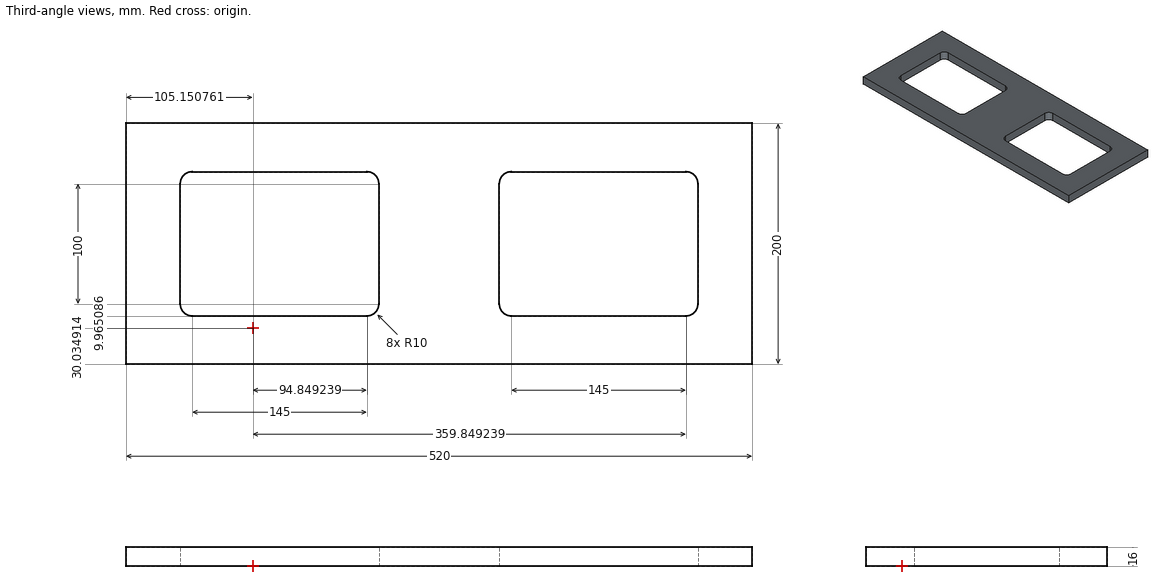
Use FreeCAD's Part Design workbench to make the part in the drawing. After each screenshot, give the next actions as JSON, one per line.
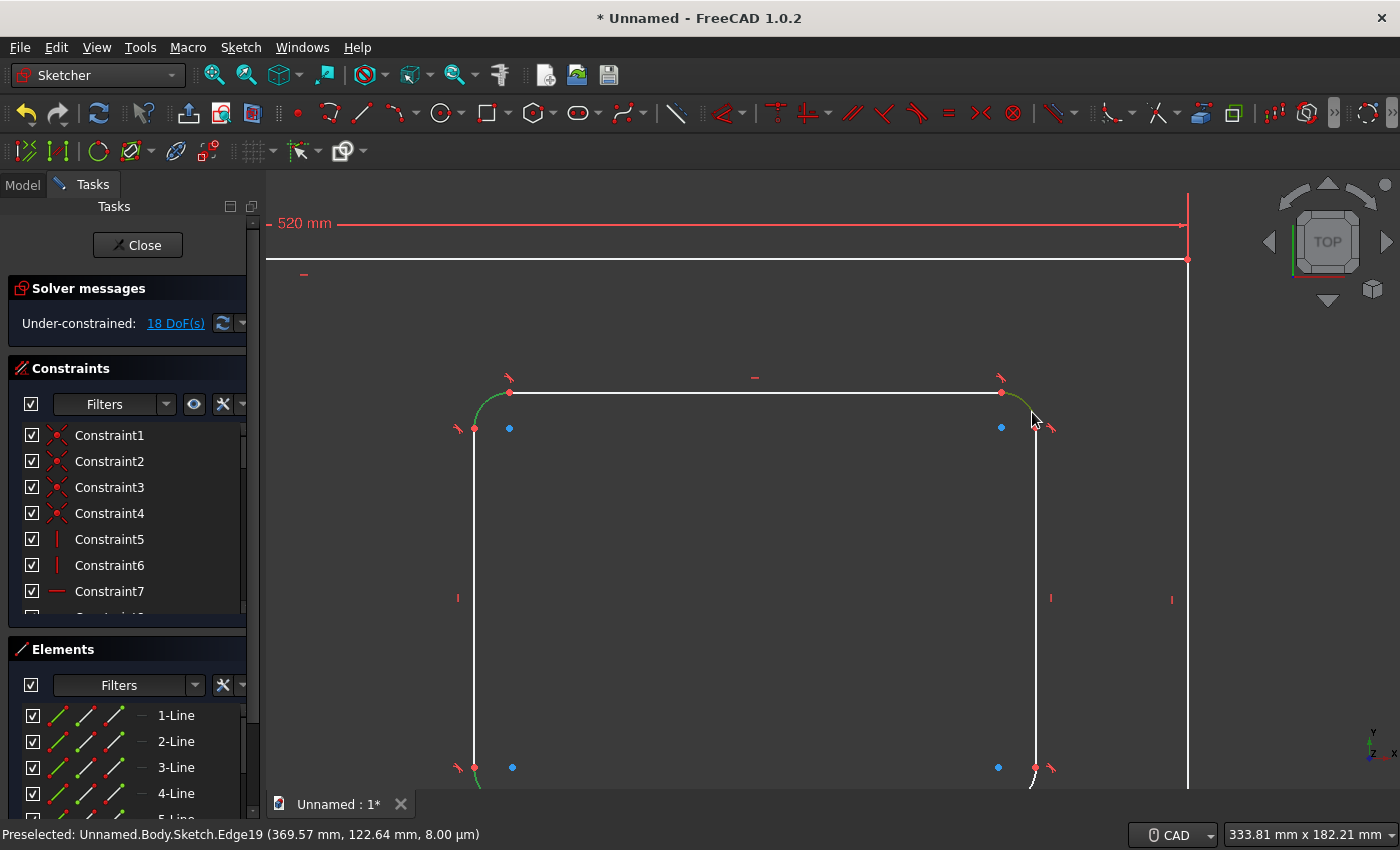
{"action": "scroll", "coordinate": [1032, 412], "scroll_direction": "down", "scroll_amount": 5}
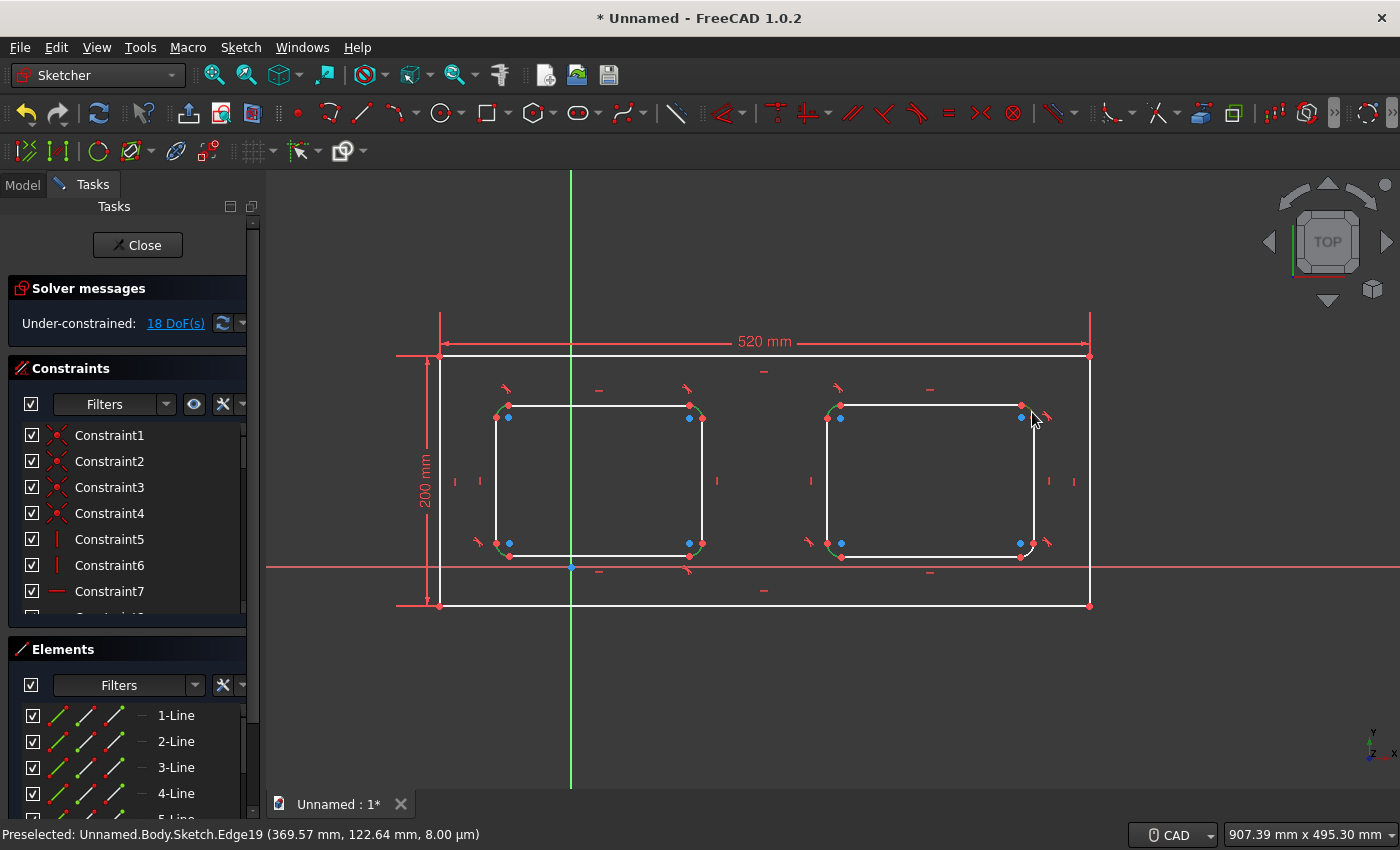
{"action": "scroll", "coordinate": [1026, 556], "scroll_direction": "up", "scroll_amount": 4}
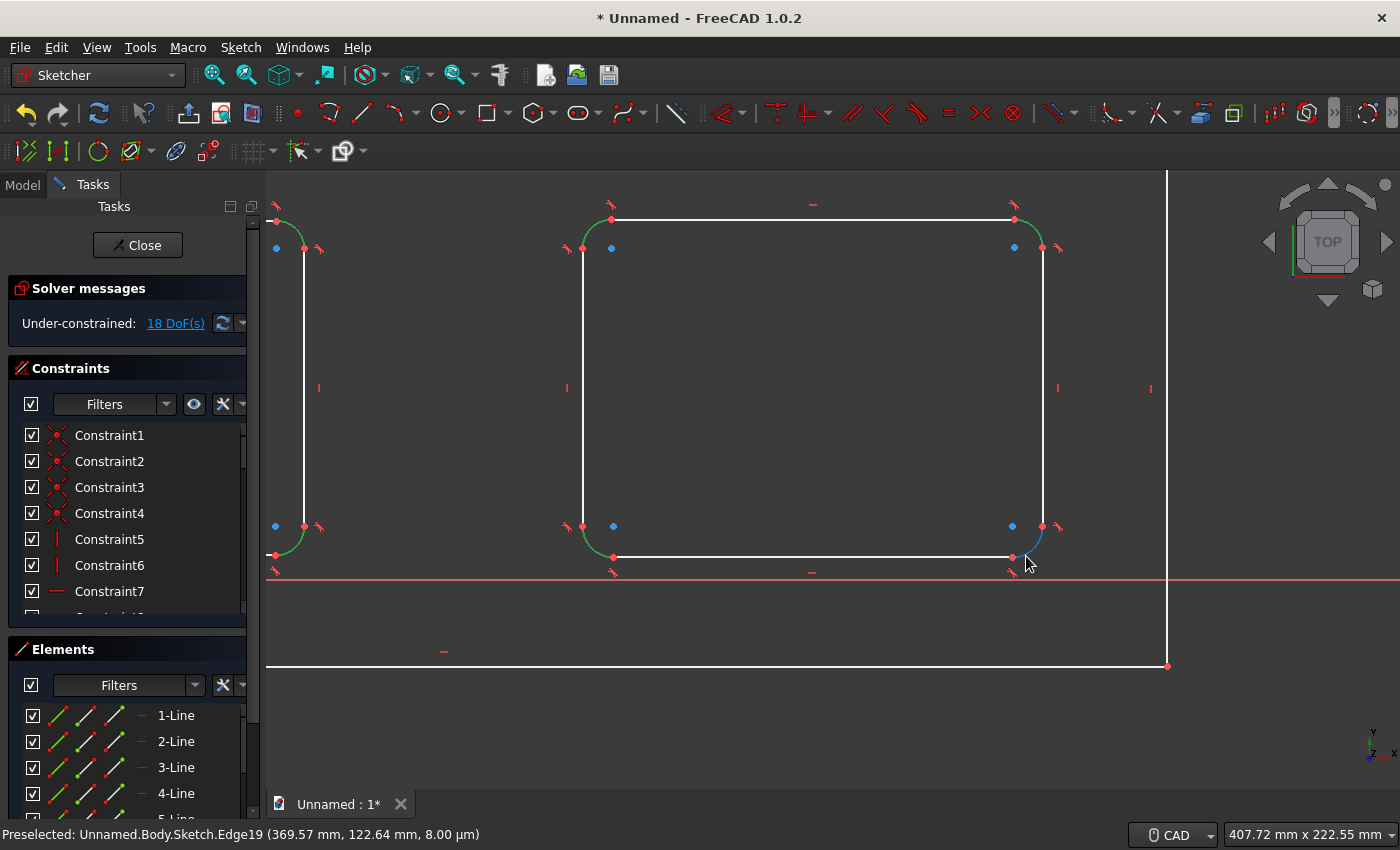
{"action": "left_click", "coordinate": [1026, 554]}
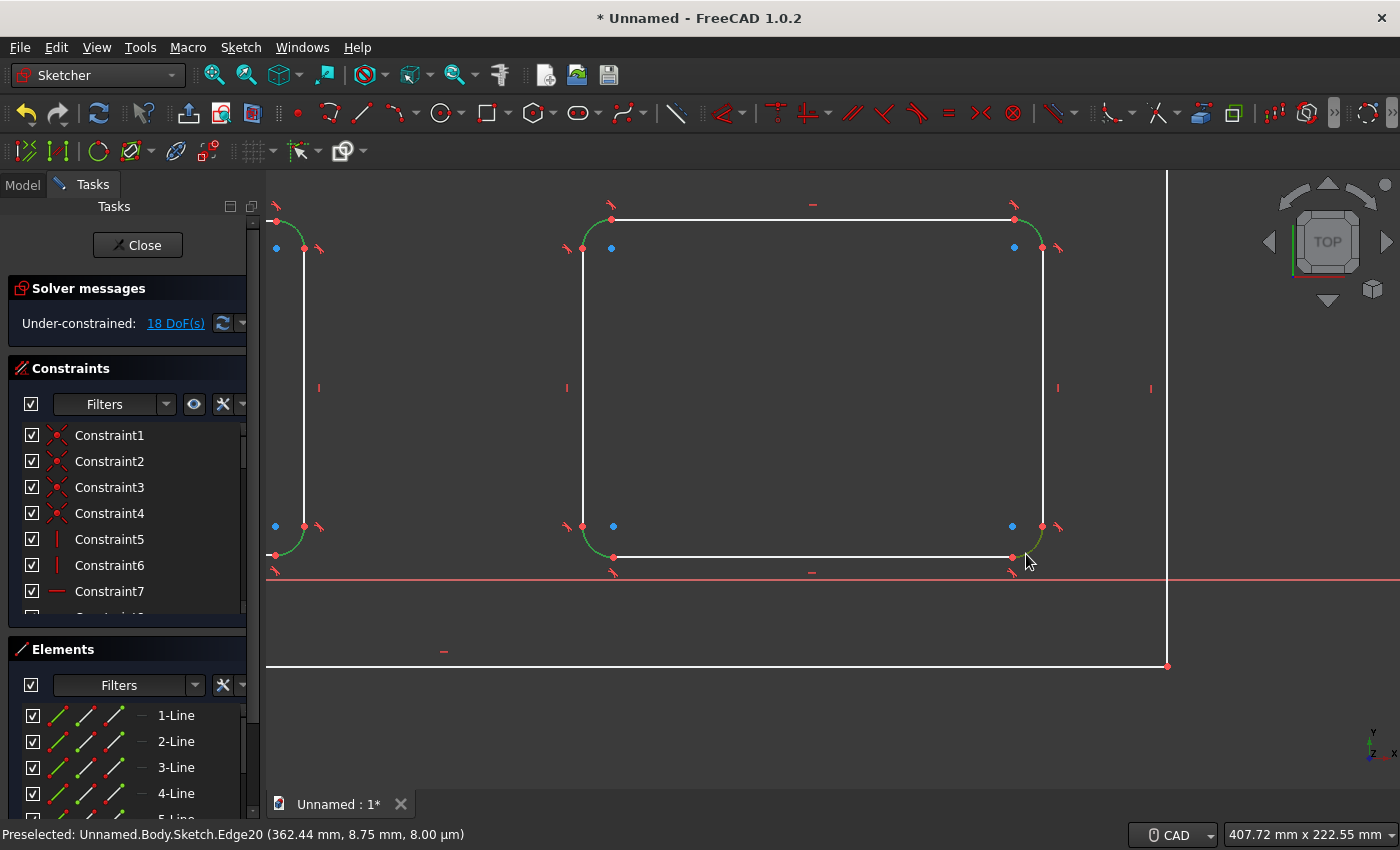
{"action": "left_click", "coordinate": [950, 114]}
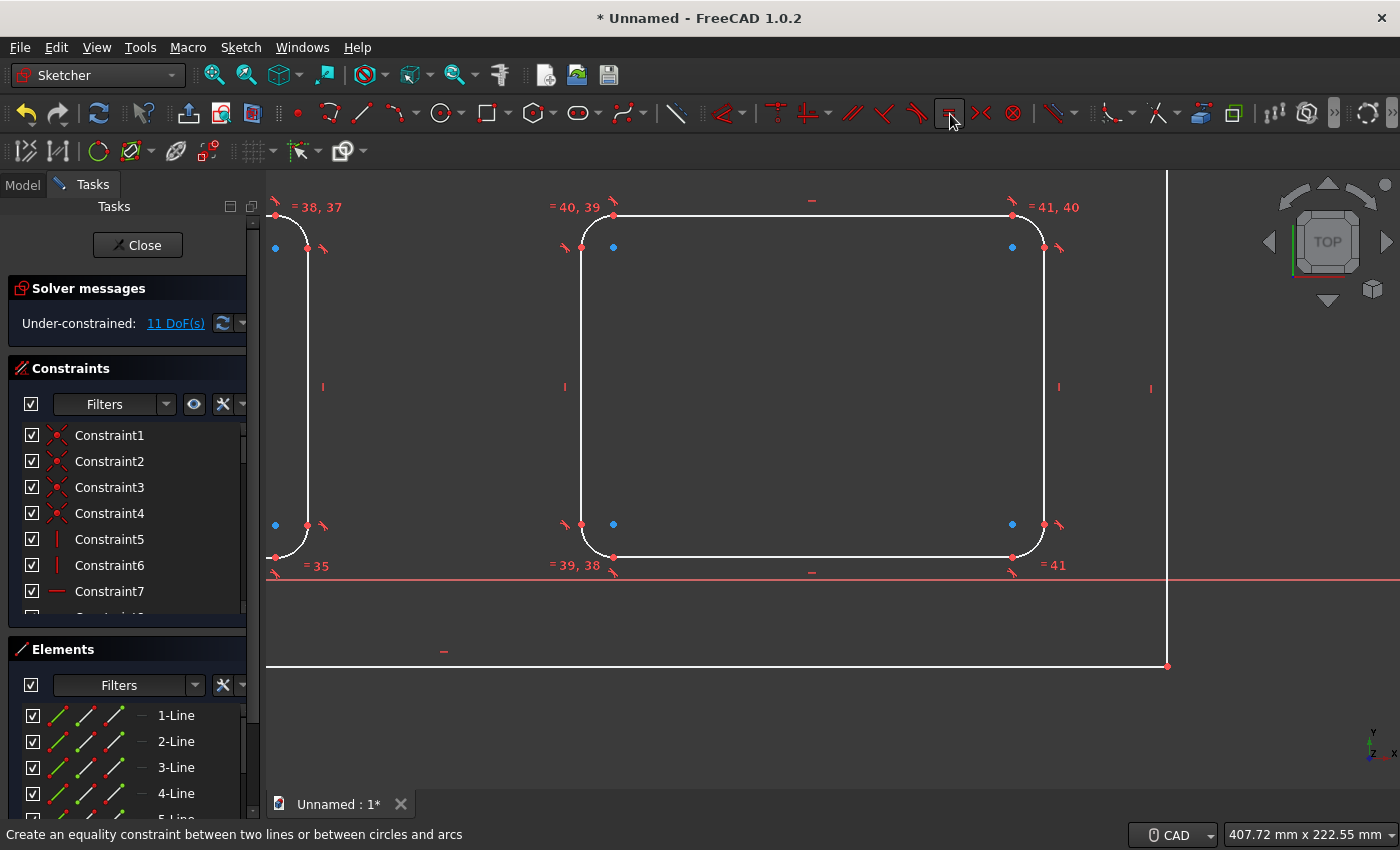
{"action": "left_click", "coordinate": [722, 114]}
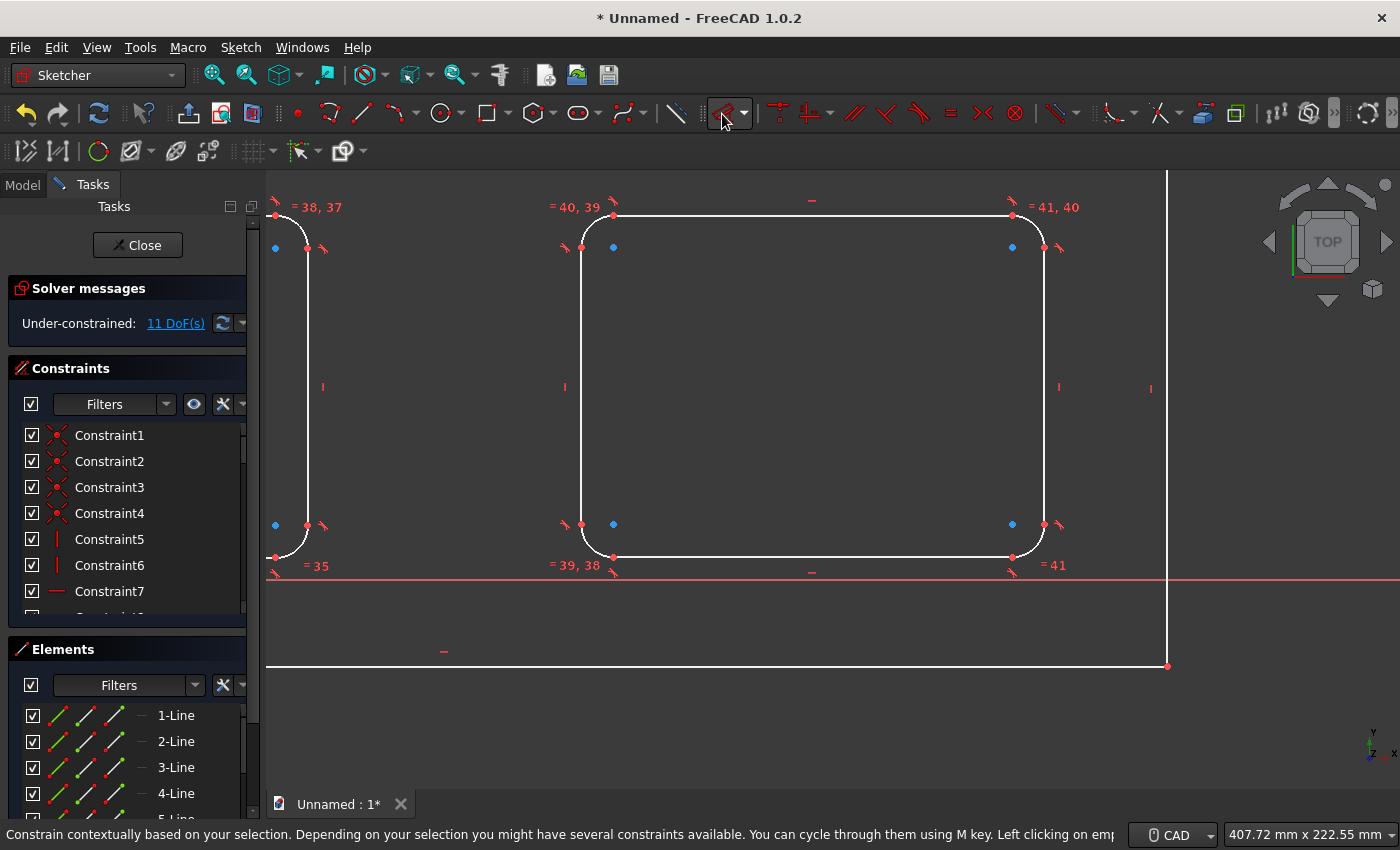
{"action": "scroll", "coordinate": [304, 540], "scroll_direction": "up", "scroll_amount": 2}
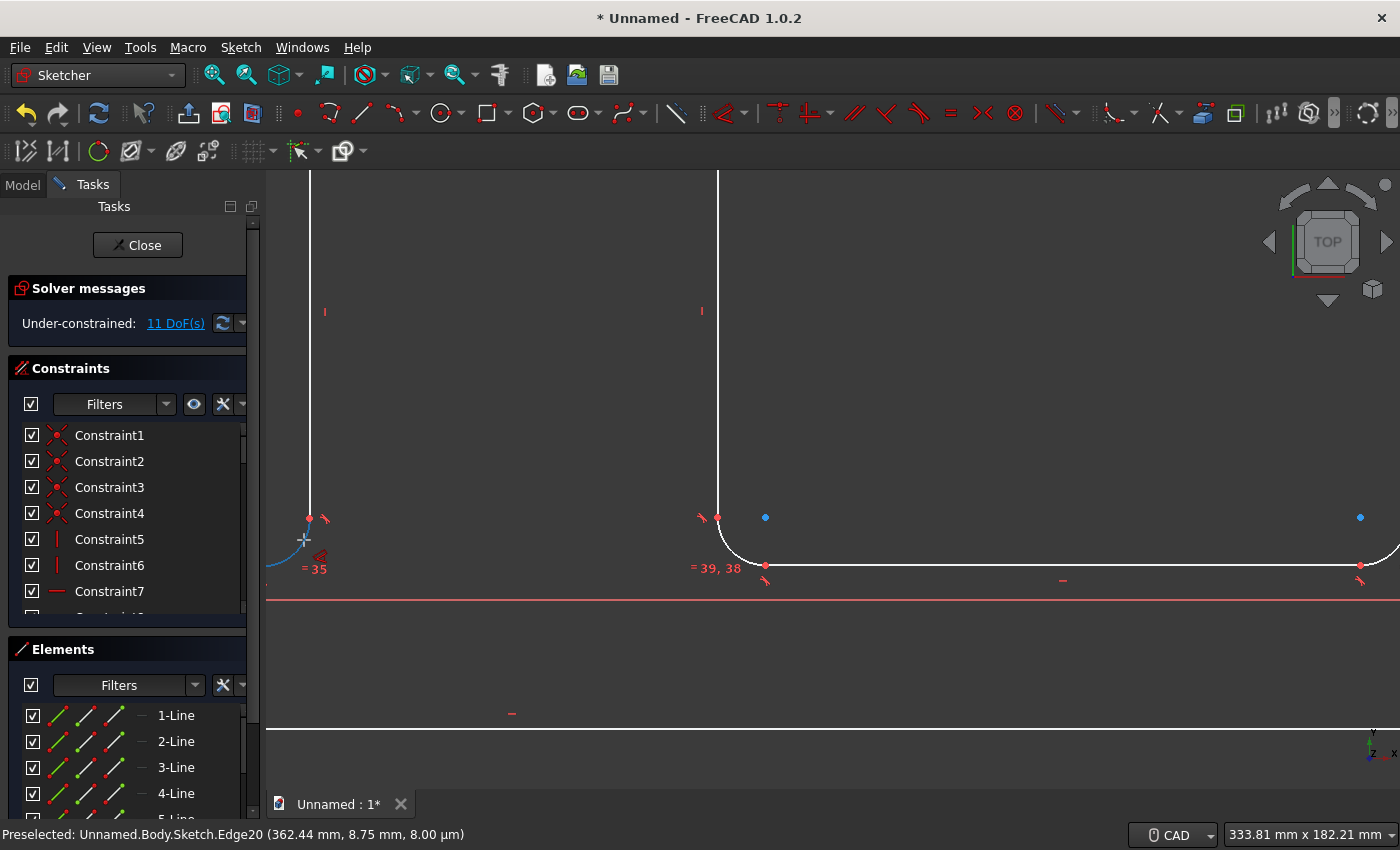
{"action": "left_click", "coordinate": [305, 540]}
{"action": "left_click", "coordinate": [334, 554]}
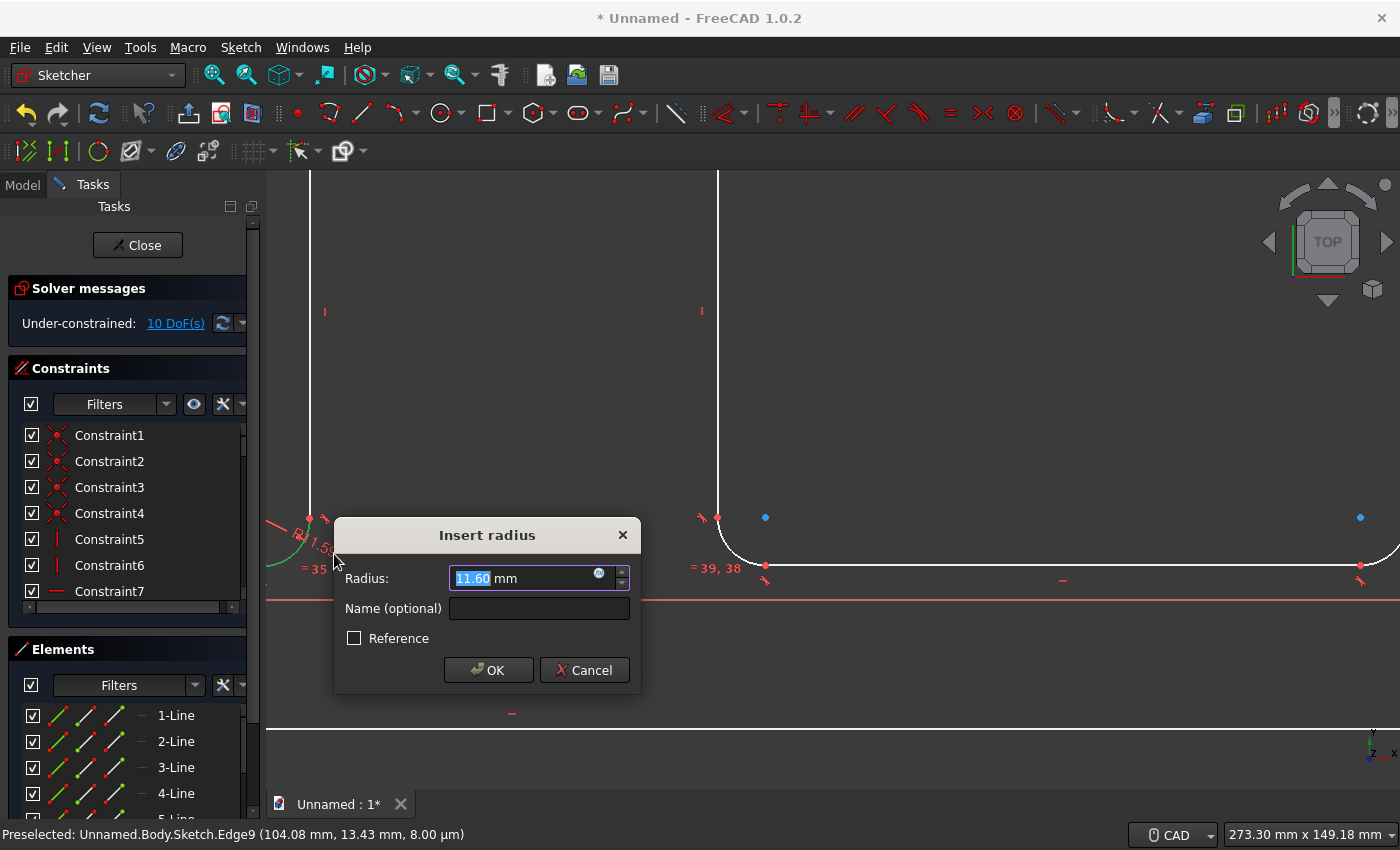
{"action": "type", "text": "10"}
{"action": "key", "text": "Return"}